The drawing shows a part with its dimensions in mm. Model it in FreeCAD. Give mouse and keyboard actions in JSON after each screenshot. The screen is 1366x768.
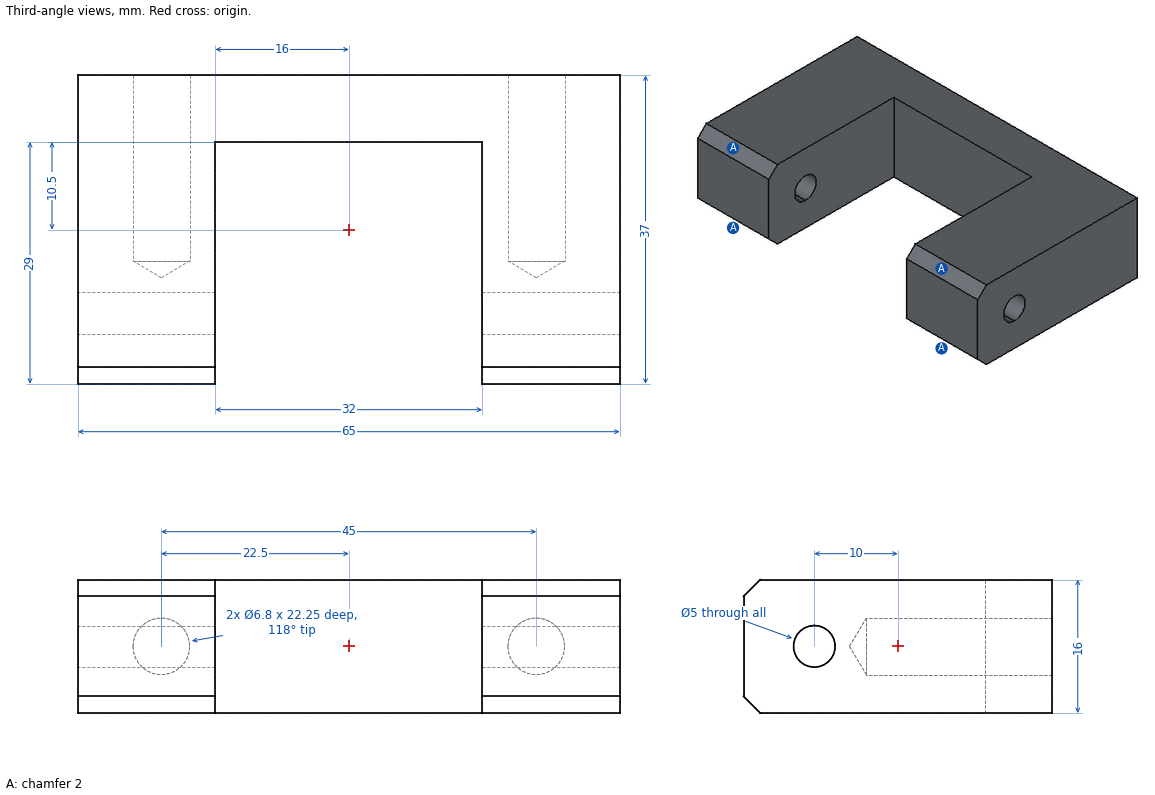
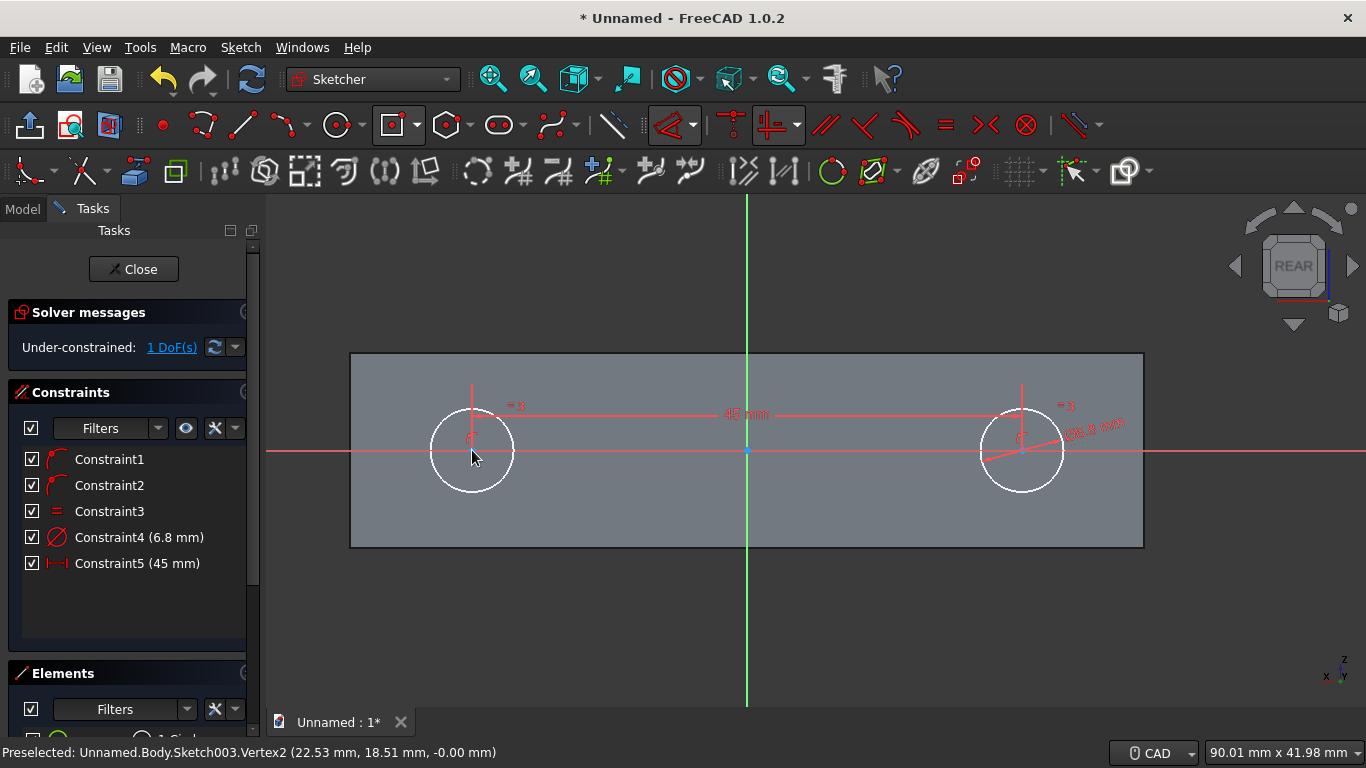
{"action": "left_click", "coordinate": [1022, 450]}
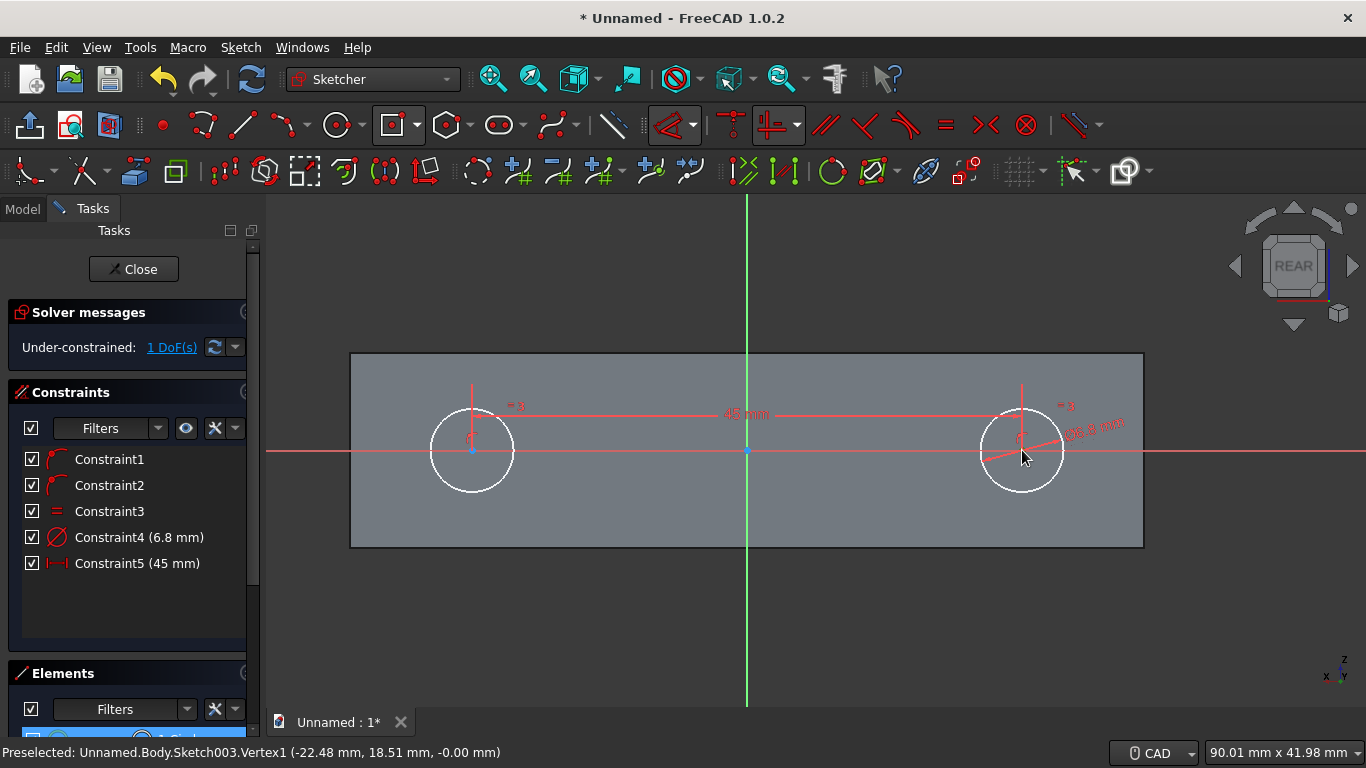
{"action": "left_click", "coordinate": [696, 126]}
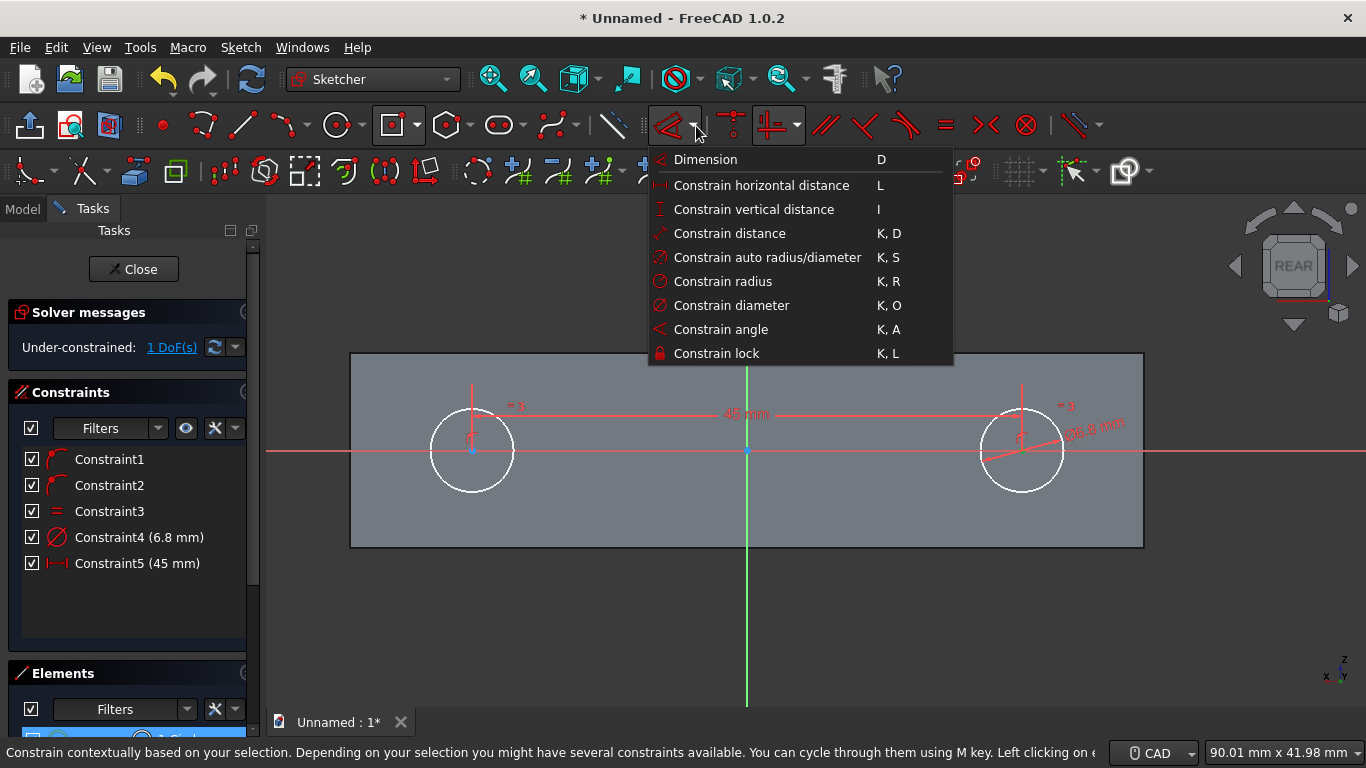
{"action": "left_click", "coordinate": [801, 185]}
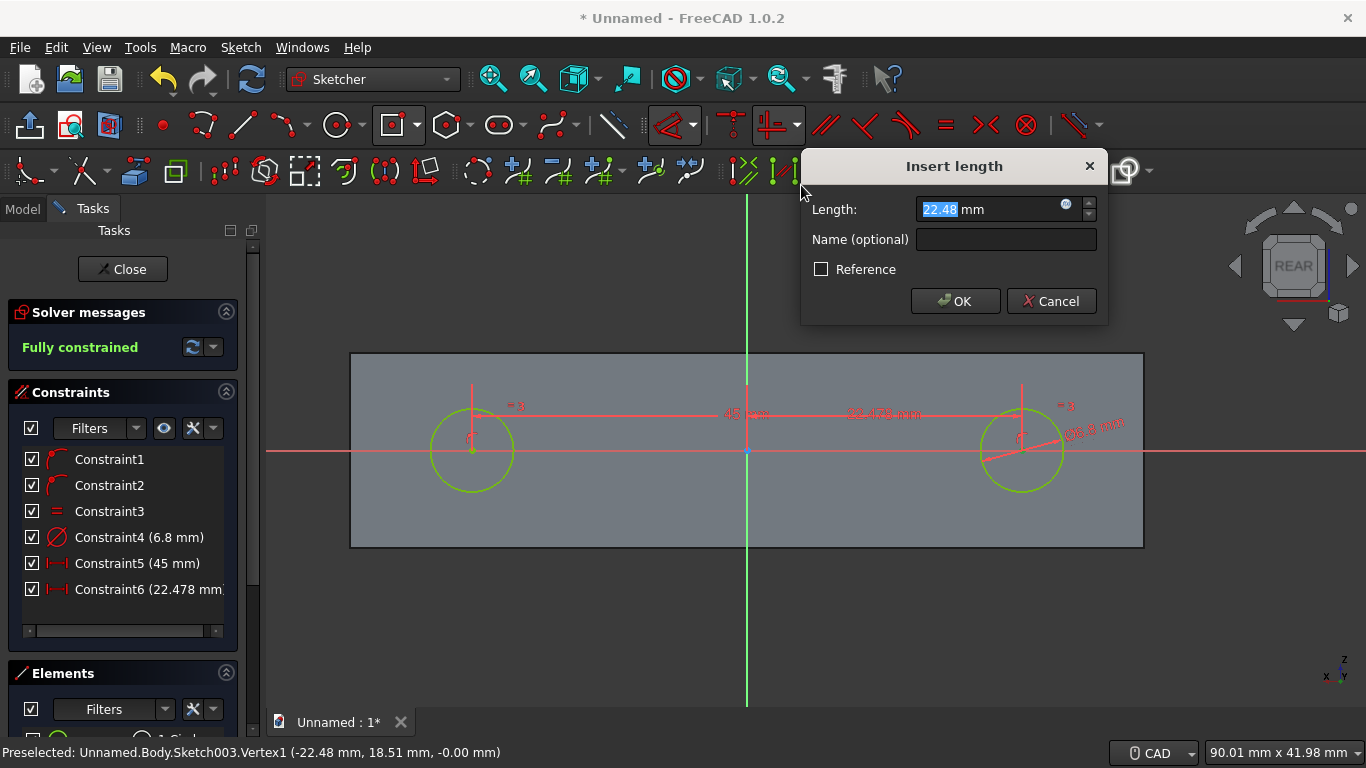
{"action": "type", "text": "22.5"}
{"action": "key", "text": "Return"}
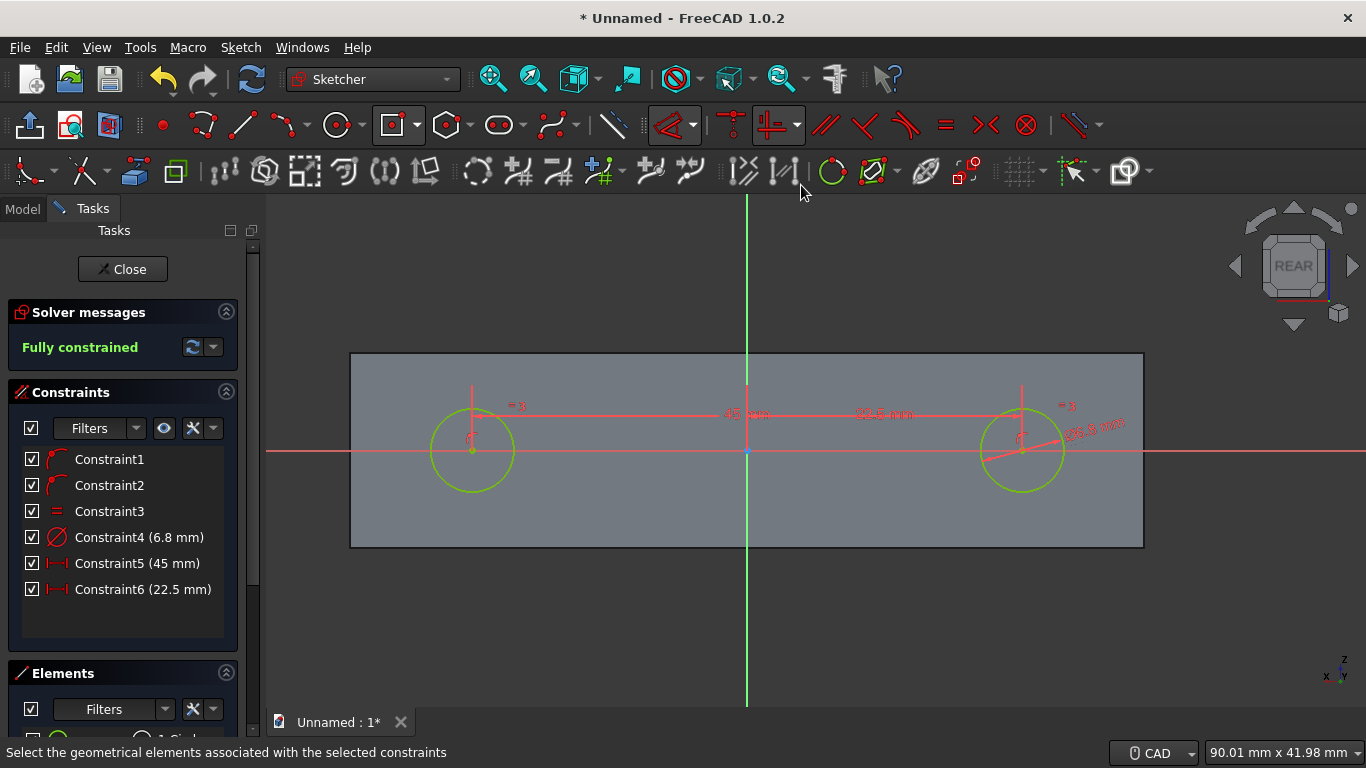
{"action": "left_click", "coordinate": [123, 269]}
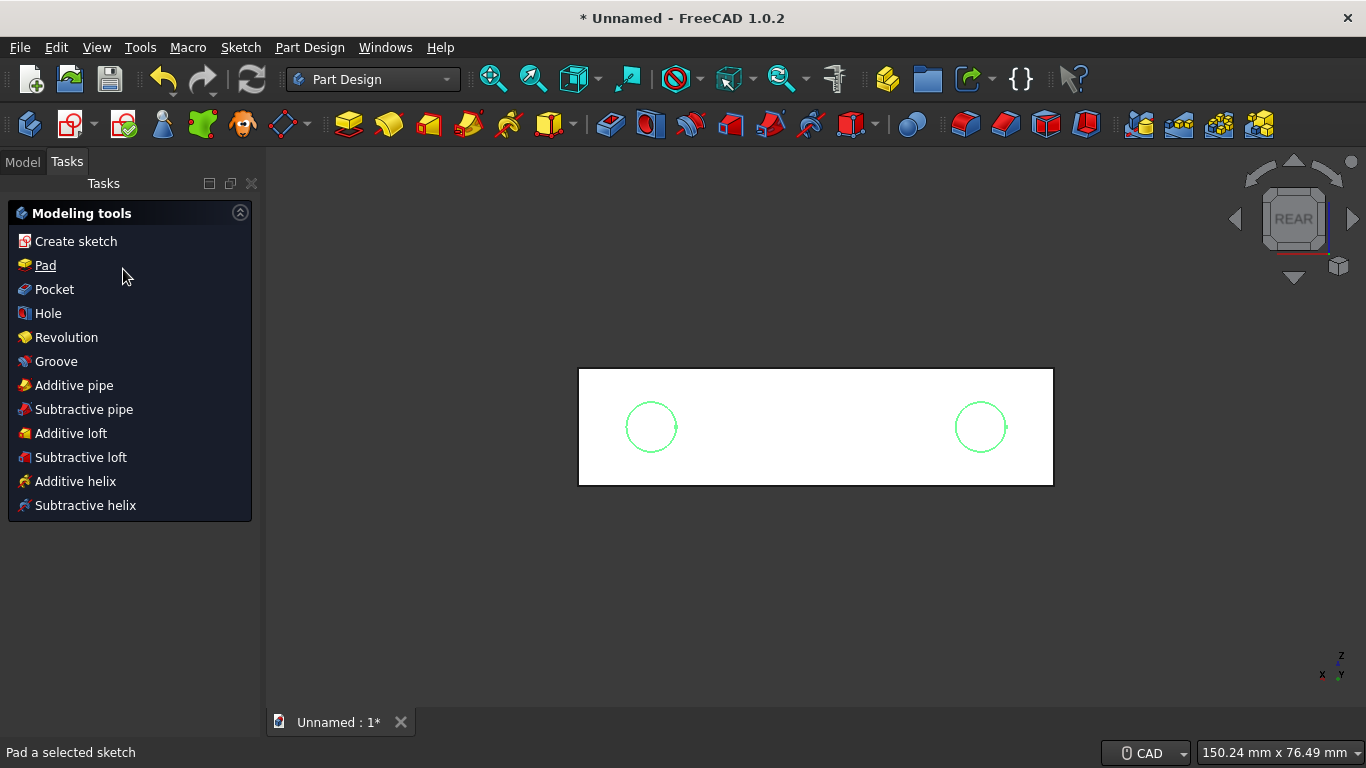
{"action": "left_click", "coordinate": [652, 124]}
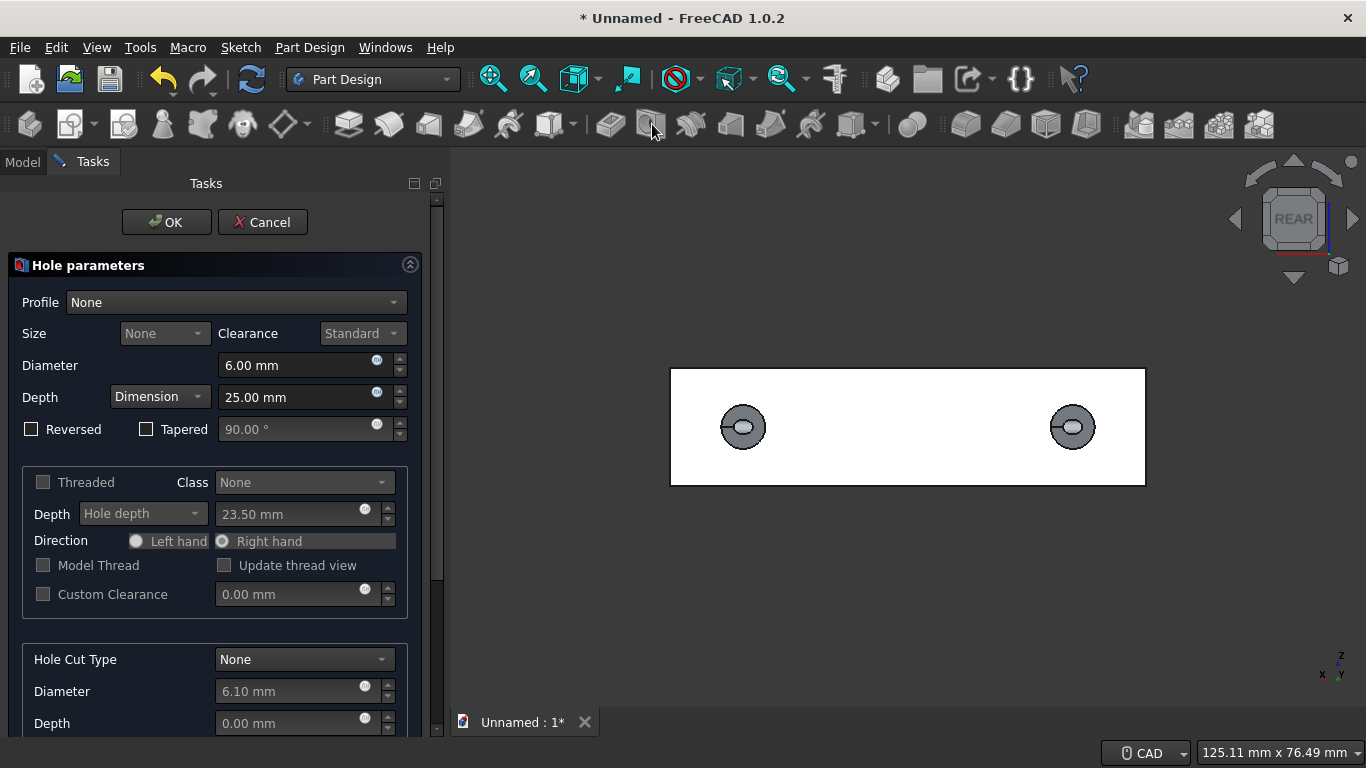
{"action": "triple_click", "coordinate": [305, 365]}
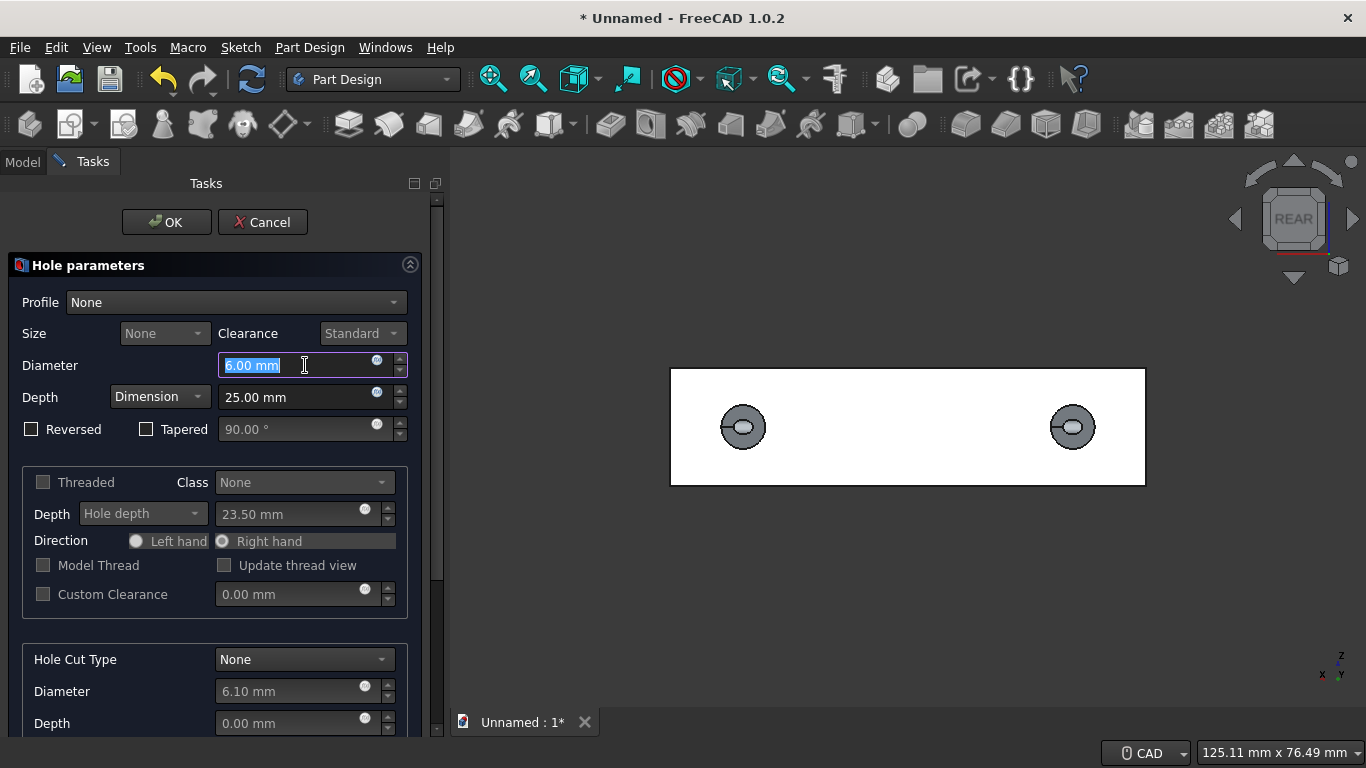
{"action": "type", "text": "6.8"}
{"action": "key", "text": "Tab"}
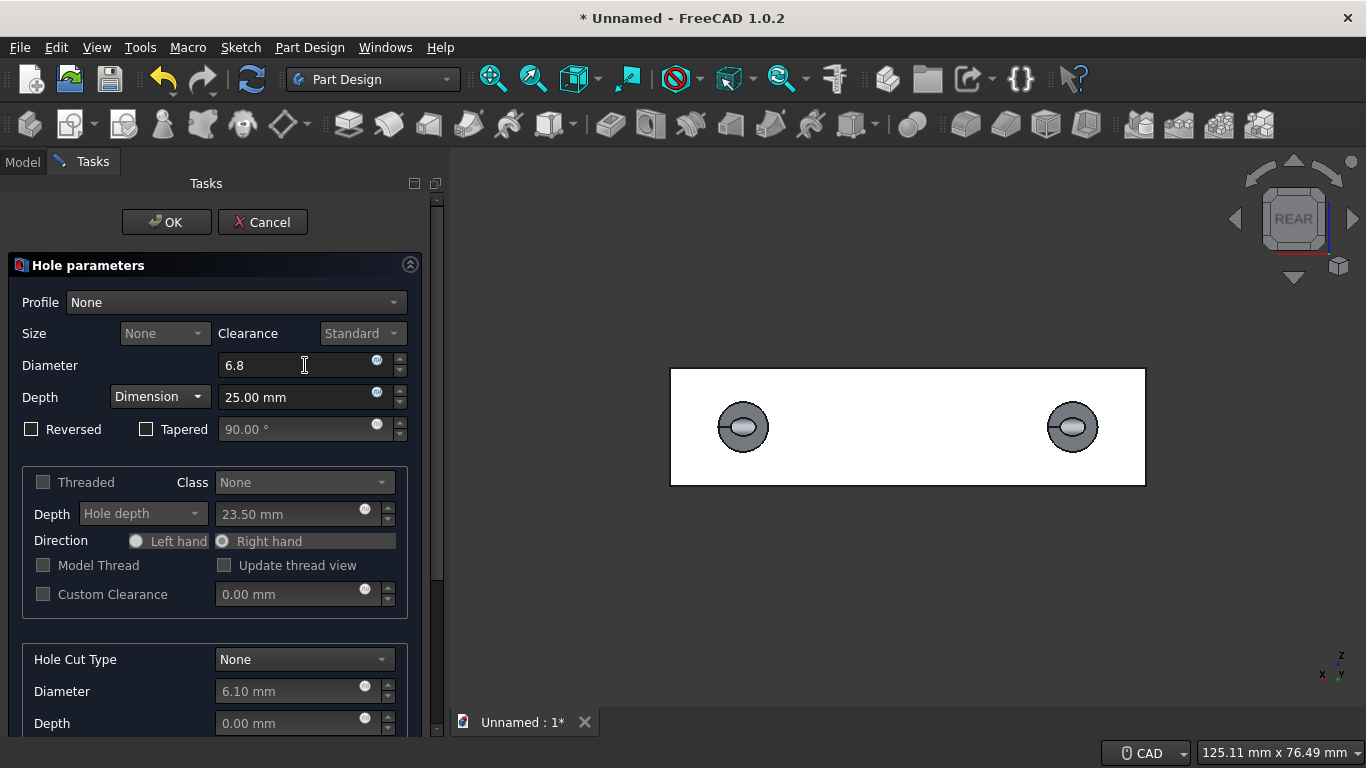
{"action": "triple_click", "coordinate": [305, 397]}